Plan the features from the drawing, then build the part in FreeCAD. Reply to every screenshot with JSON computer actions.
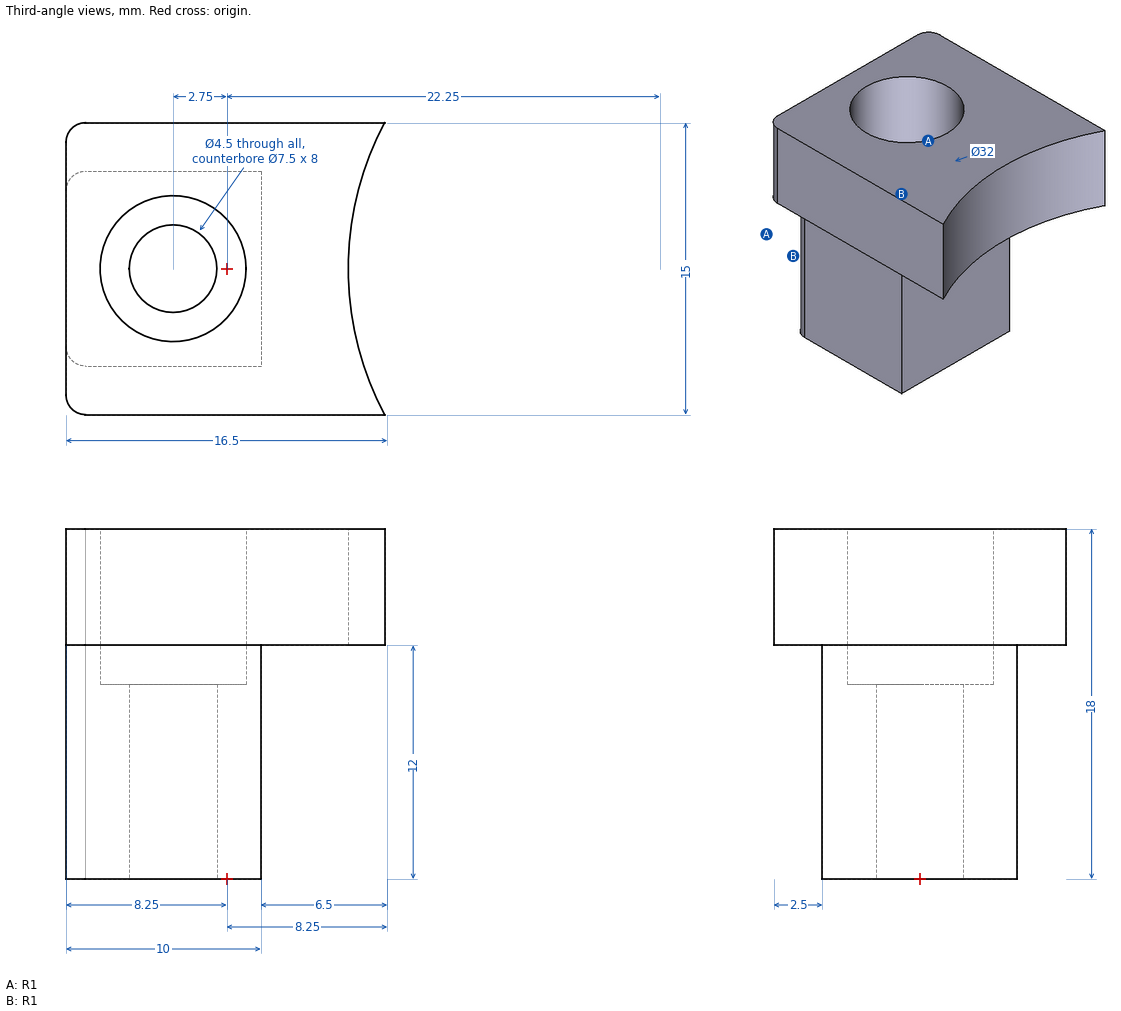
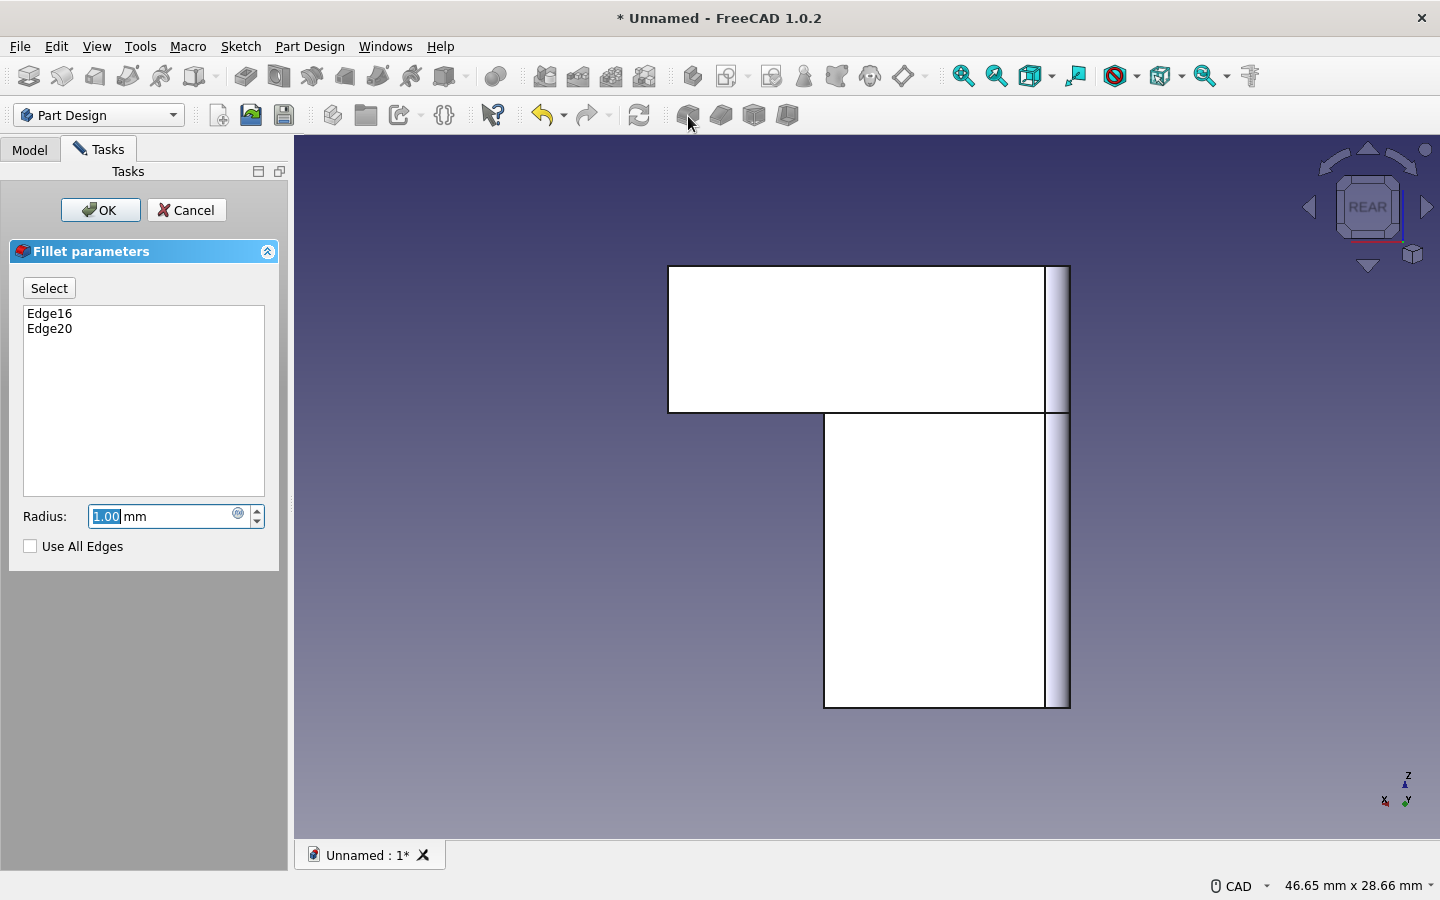
{"action": "type", "text": "1"}
{"action": "key", "text": "Tab"}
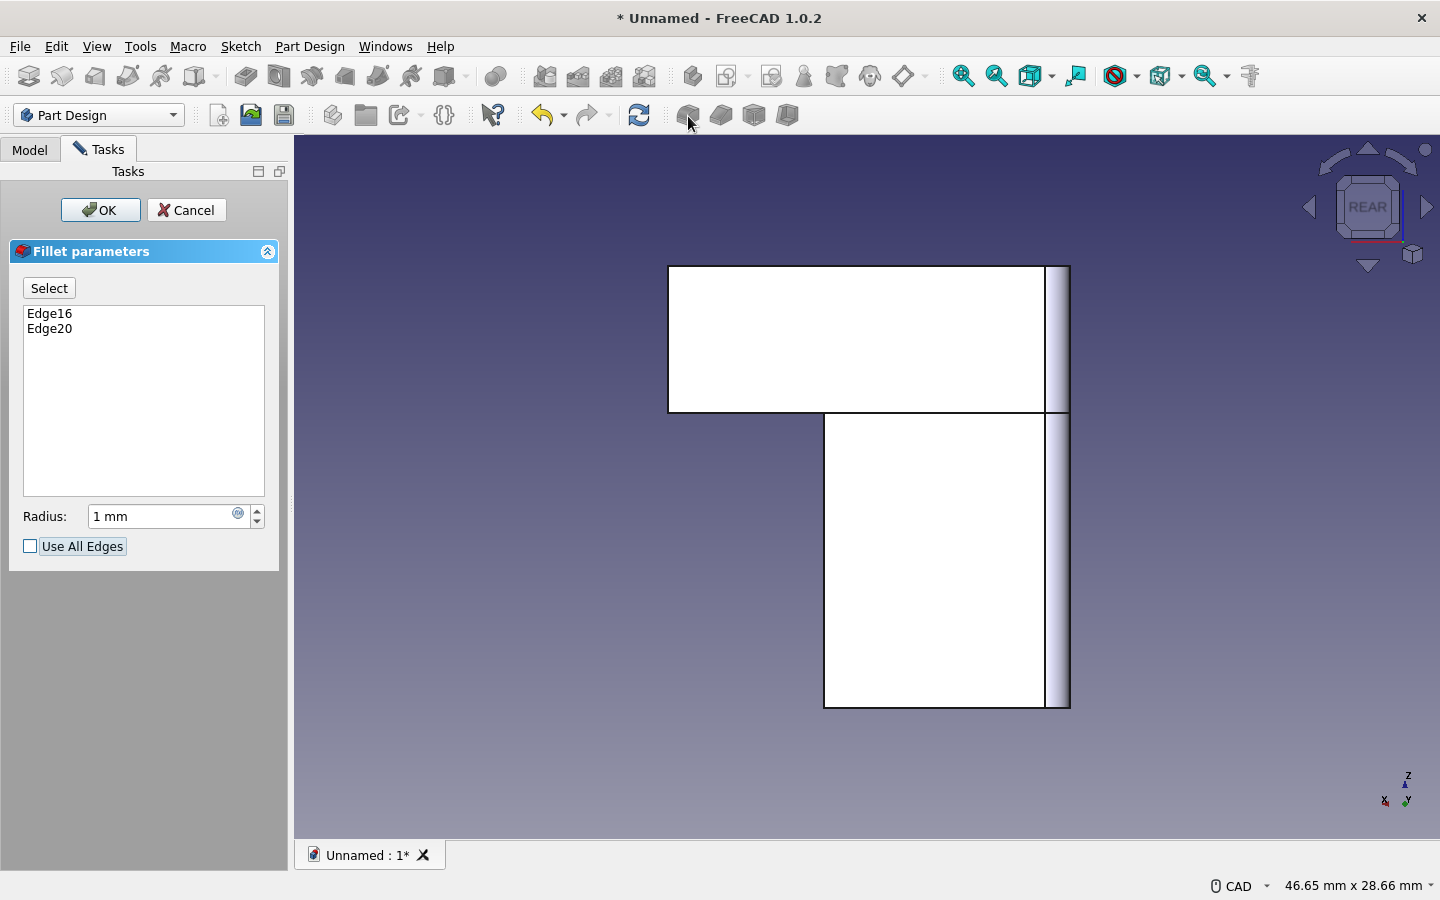
{"action": "left_click", "coordinate": [101, 210]}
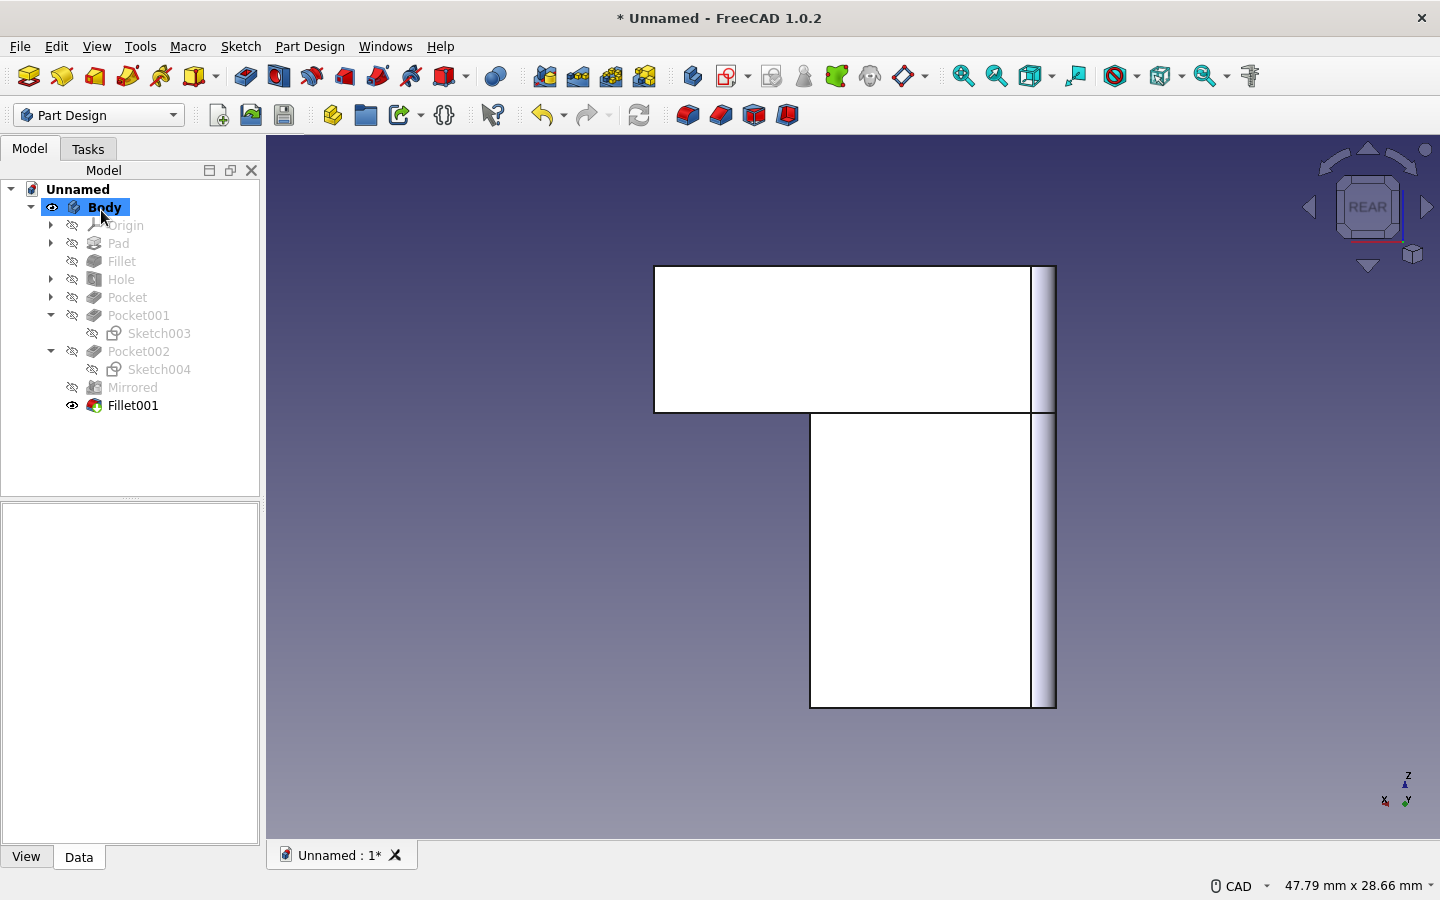
{"action": "key", "text": "0"}